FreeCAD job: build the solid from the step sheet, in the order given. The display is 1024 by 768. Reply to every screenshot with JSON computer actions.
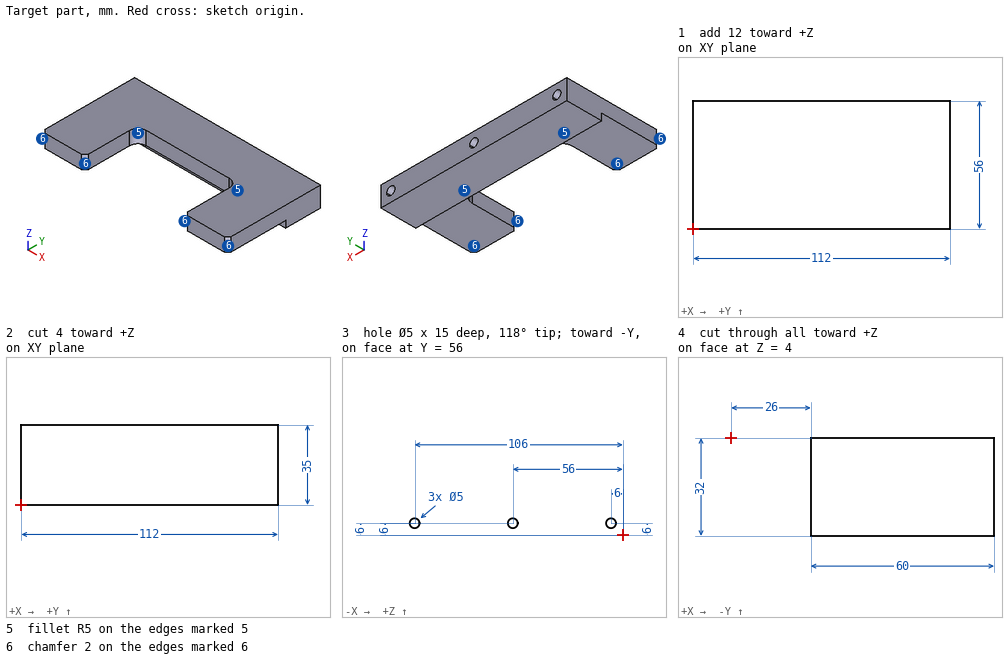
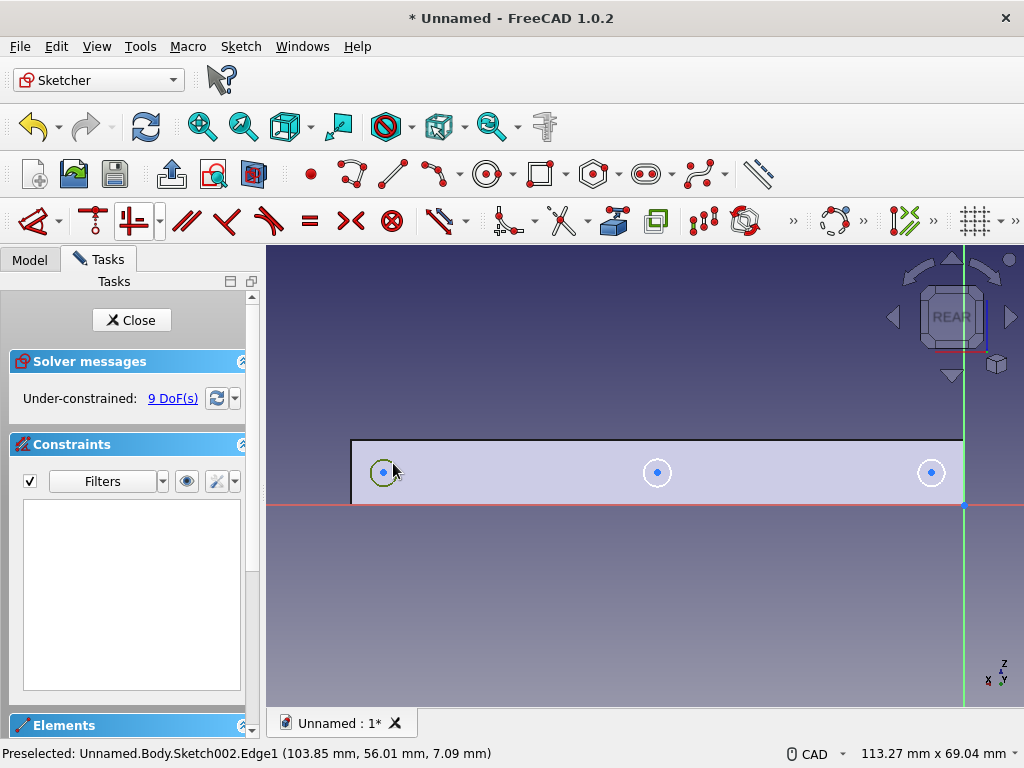
{"action": "scroll", "coordinate": [760, 464], "scroll_direction": "up", "scroll_amount": 3}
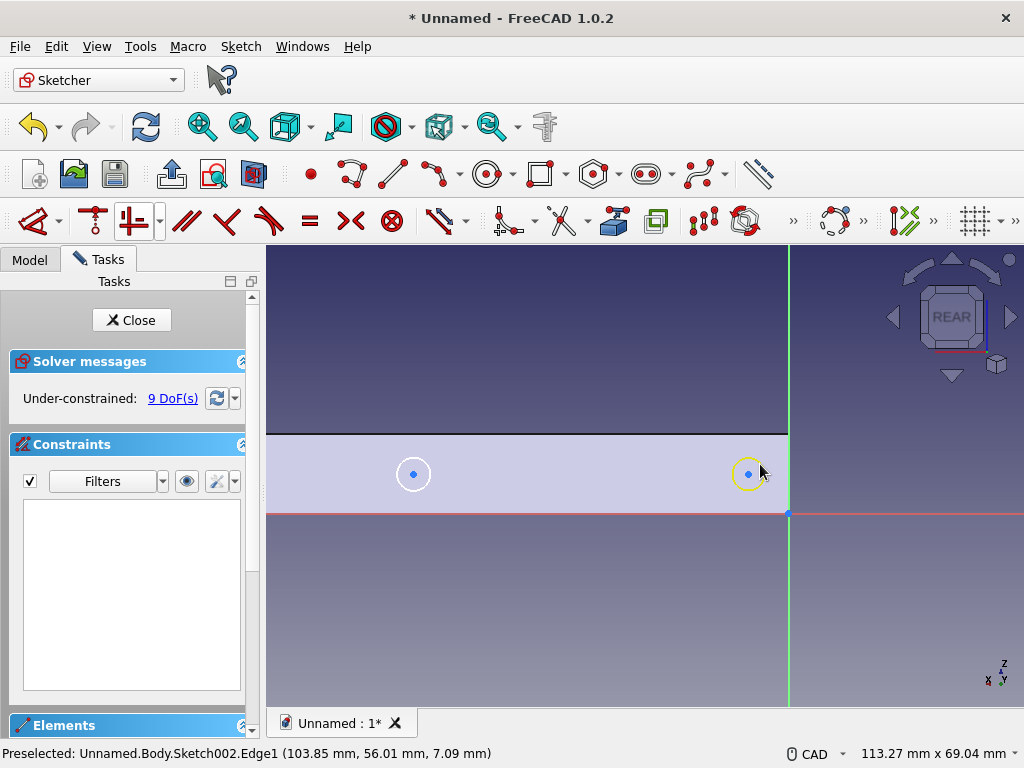
{"action": "left_click", "coordinate": [760, 463]}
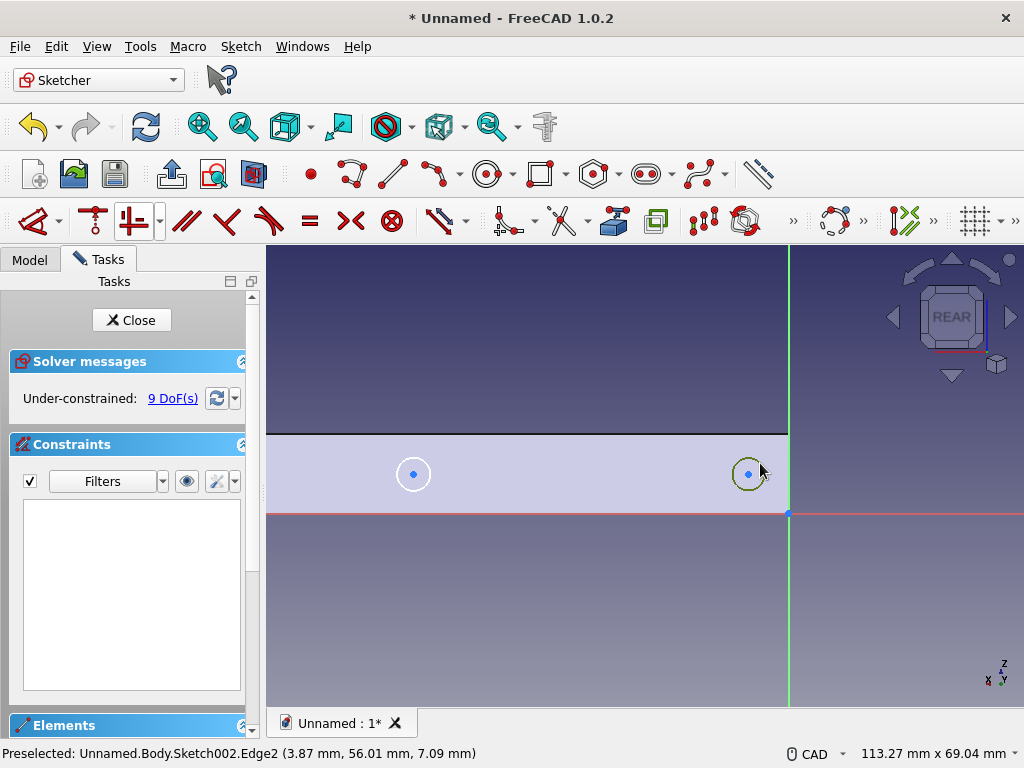
{"action": "left_click", "coordinate": [425, 463]}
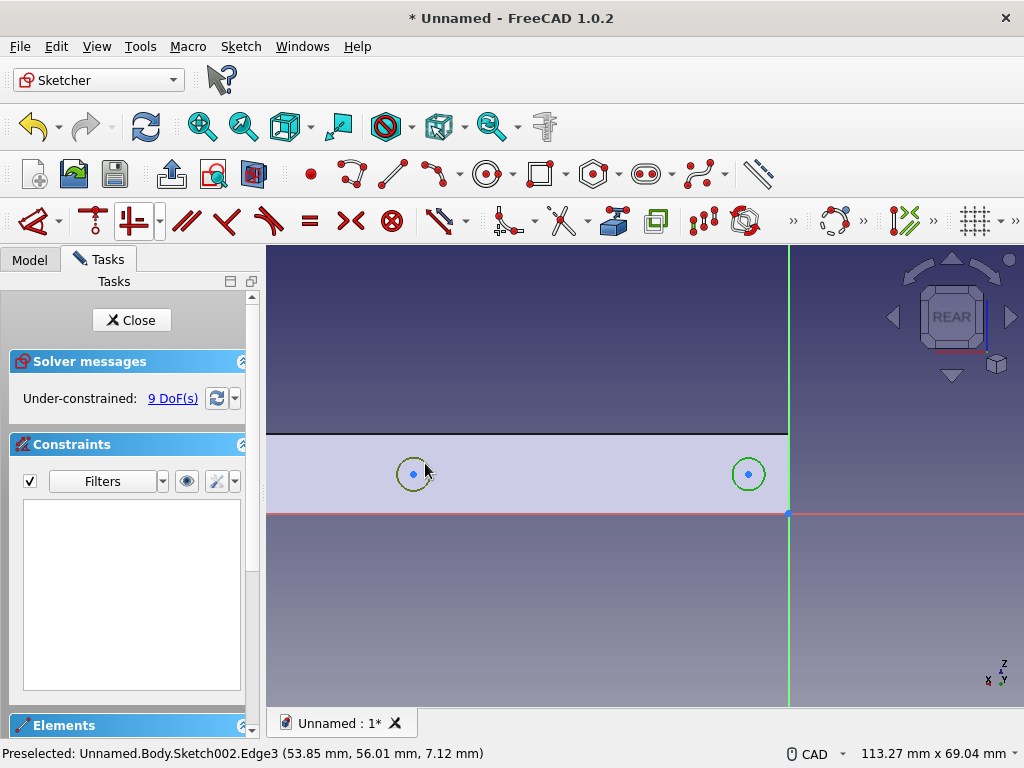
{"action": "left_click", "coordinate": [310, 222]}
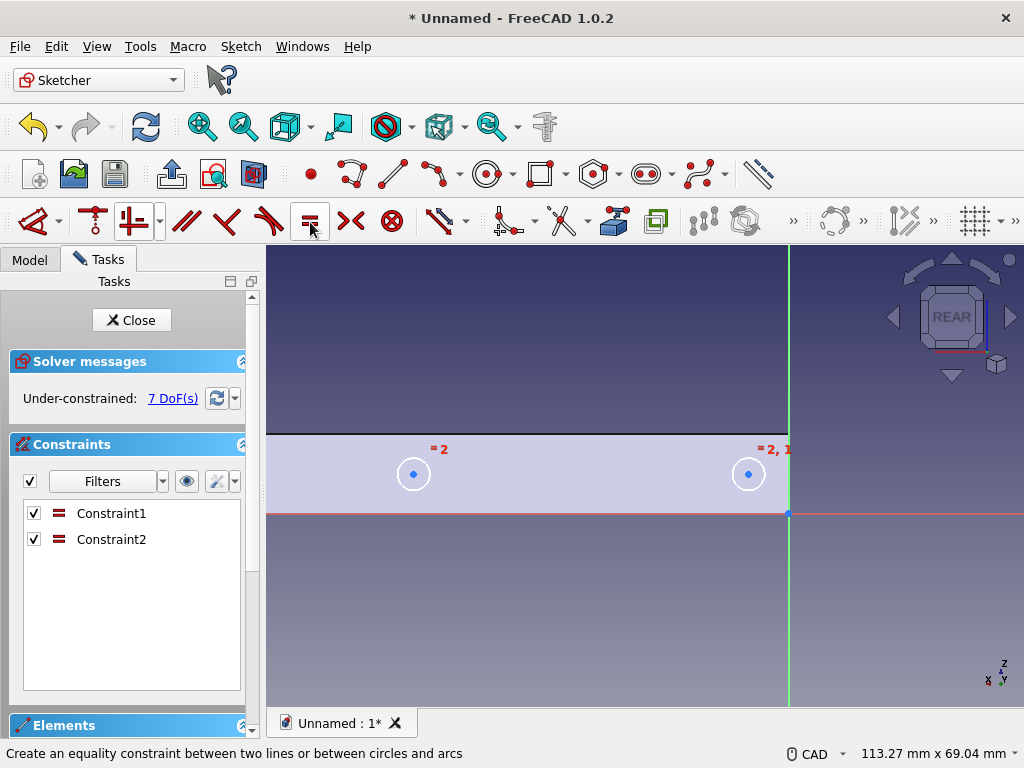
{"action": "left_click", "coordinate": [32, 222]}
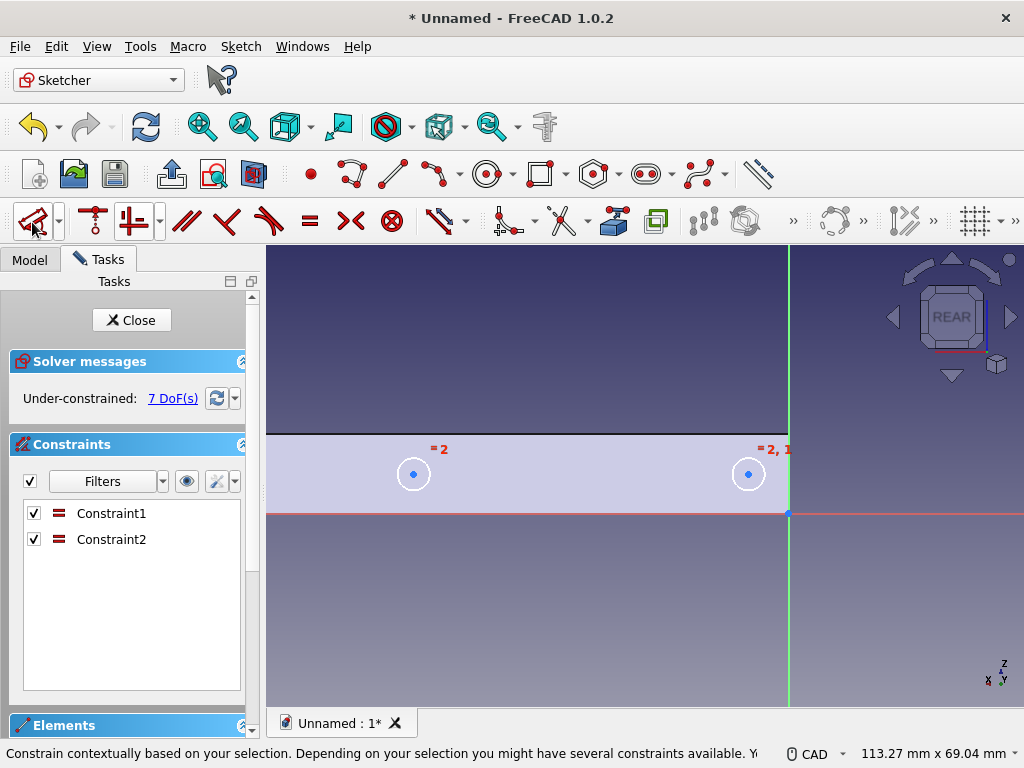
{"action": "scroll", "coordinate": [760, 464], "scroll_direction": "down", "scroll_amount": 3}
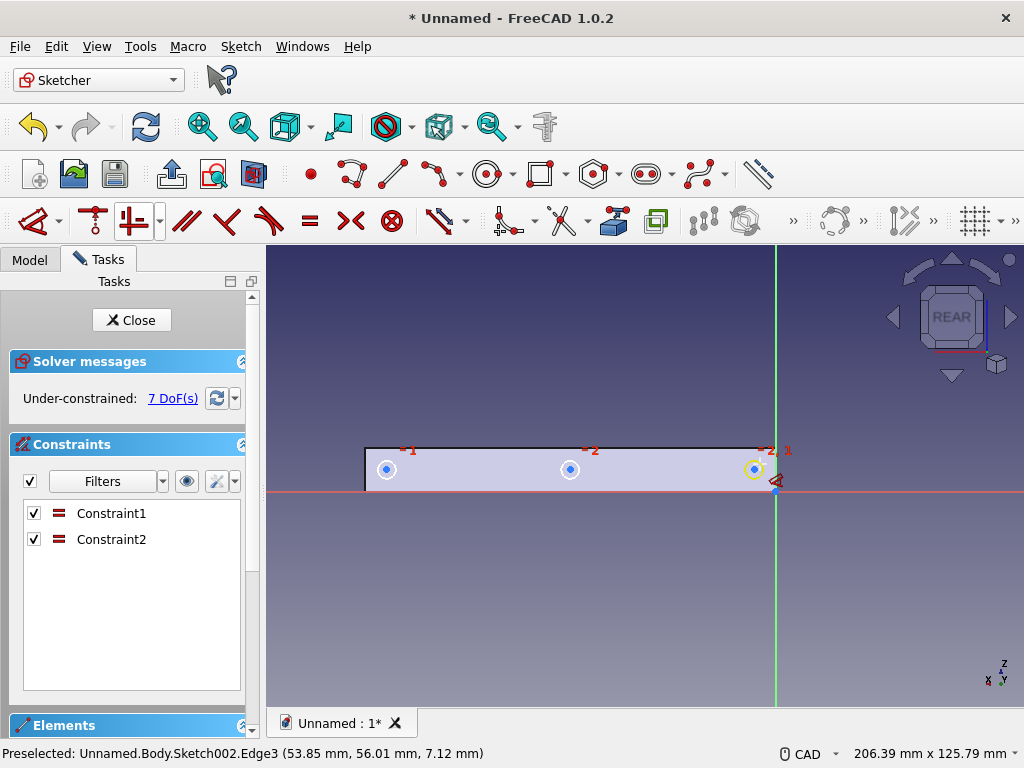
{"action": "scroll", "coordinate": [393, 464], "scroll_direction": "up", "scroll_amount": 4}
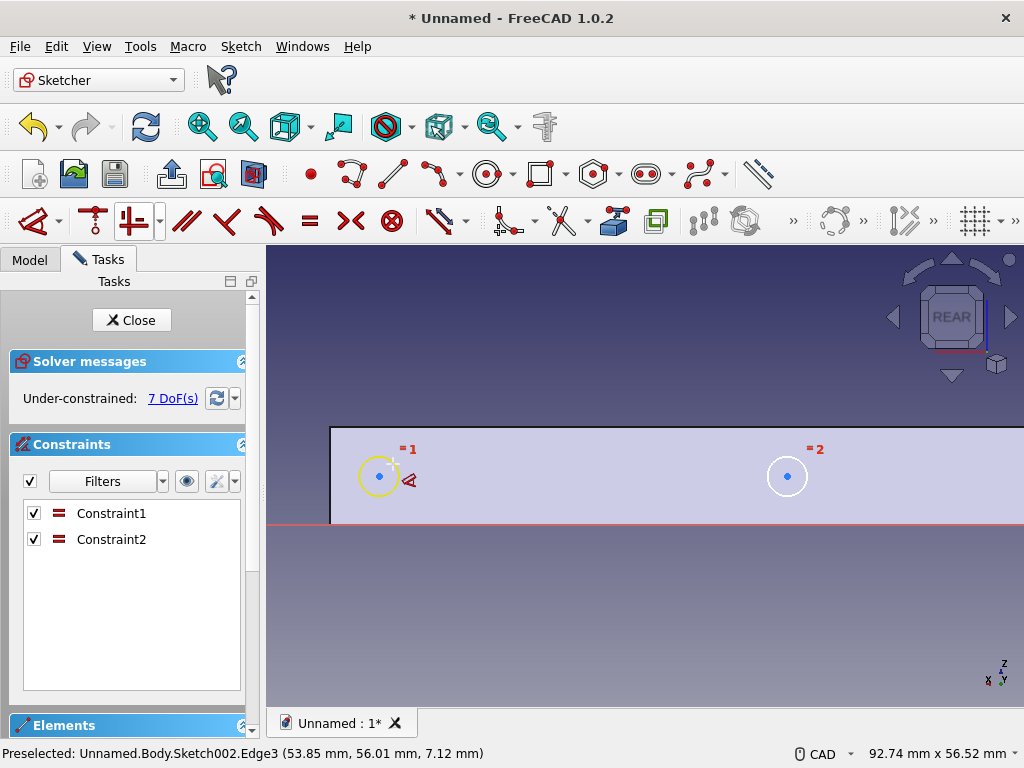
{"action": "left_click", "coordinate": [393, 462]}
{"action": "left_click", "coordinate": [415, 439]}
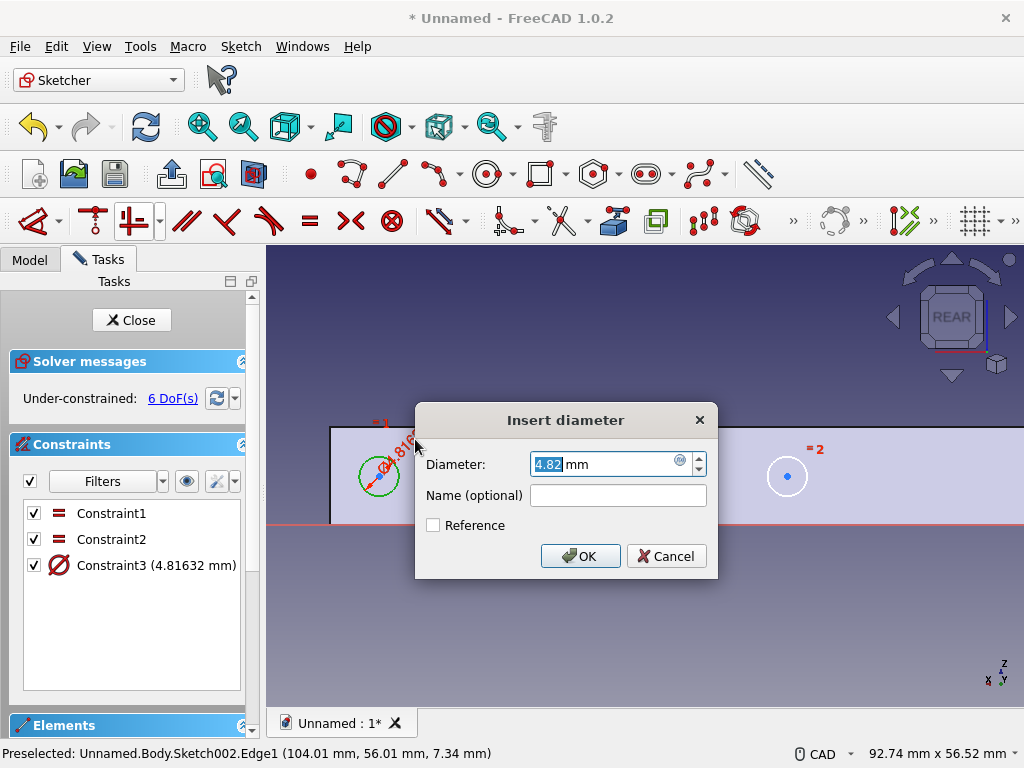
{"action": "type", "text": "5"}
{"action": "key", "text": "Return"}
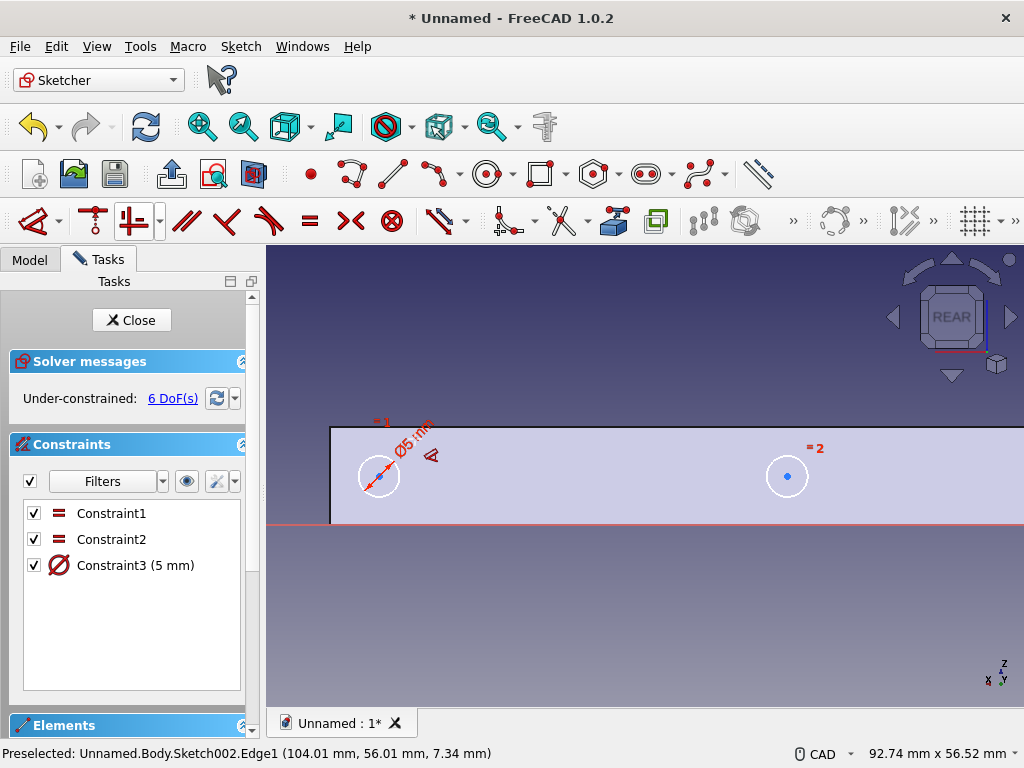
{"action": "left_click", "coordinate": [379, 476]}
{"action": "left_click", "coordinate": [345, 501]}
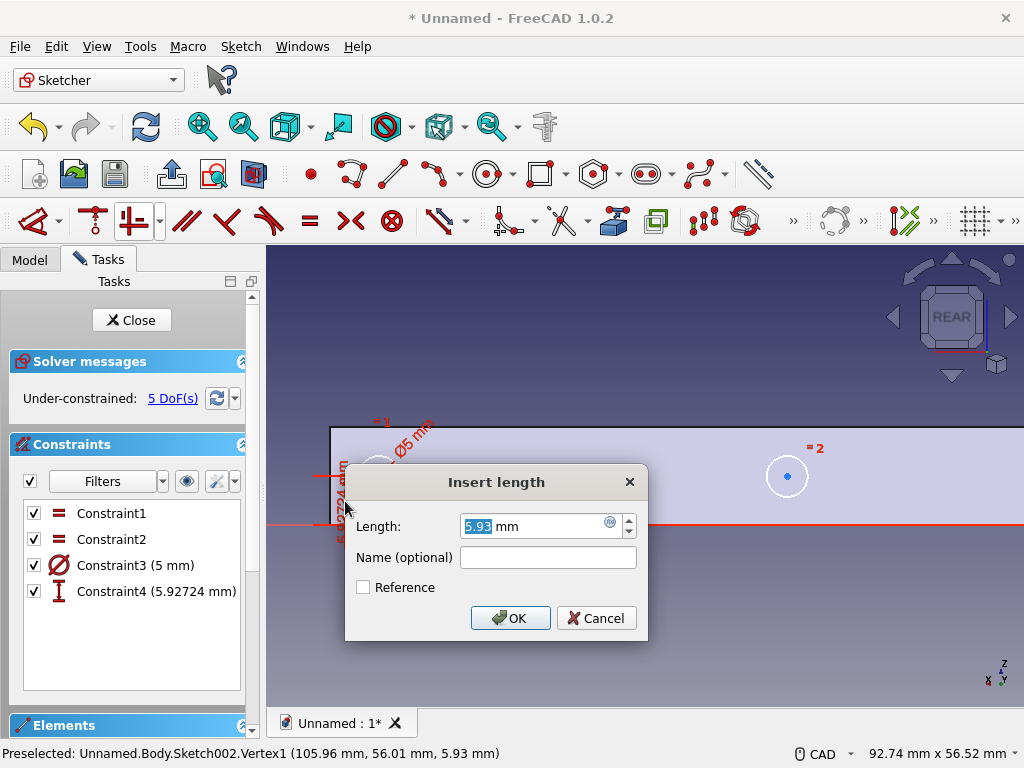
{"action": "type", "text": "6"}
{"action": "key", "text": "Return"}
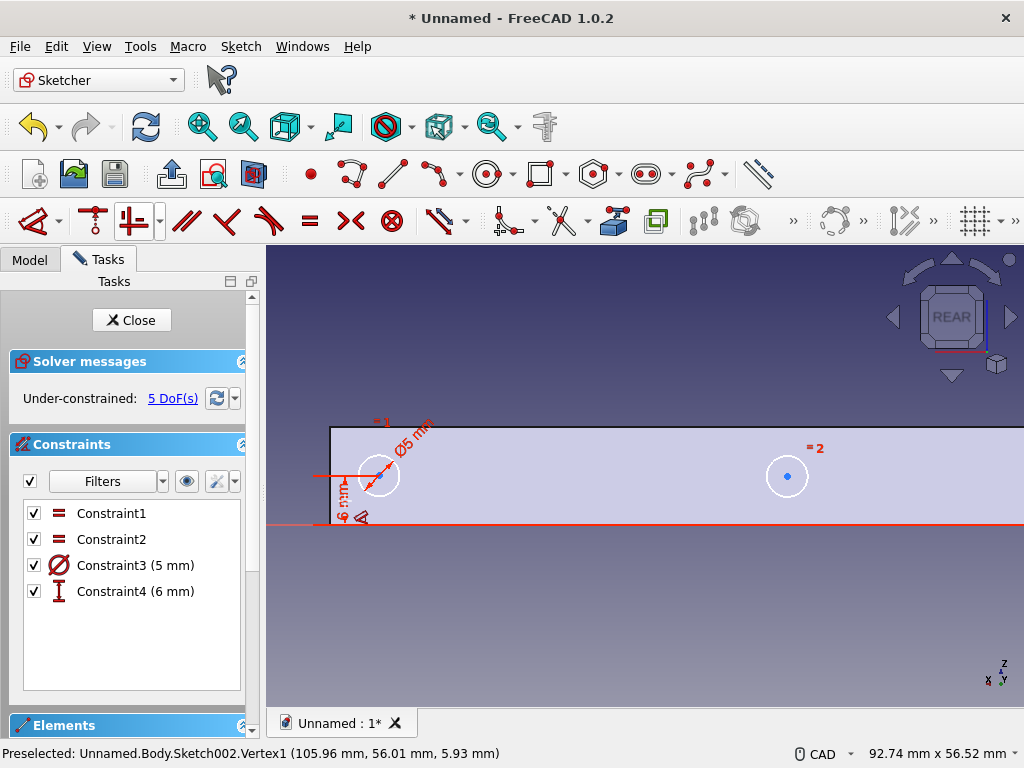
{"action": "scroll", "coordinate": [393, 464], "scroll_direction": "down", "scroll_amount": 4}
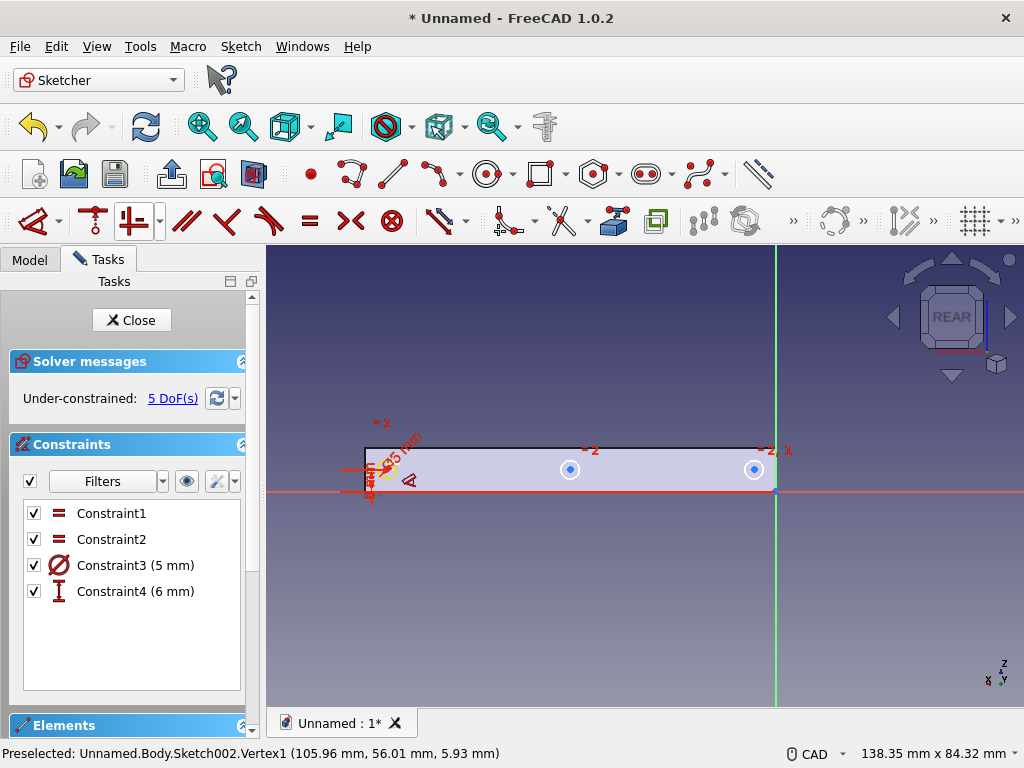
{"action": "scroll", "coordinate": [754, 470], "scroll_direction": "up", "scroll_amount": 3}